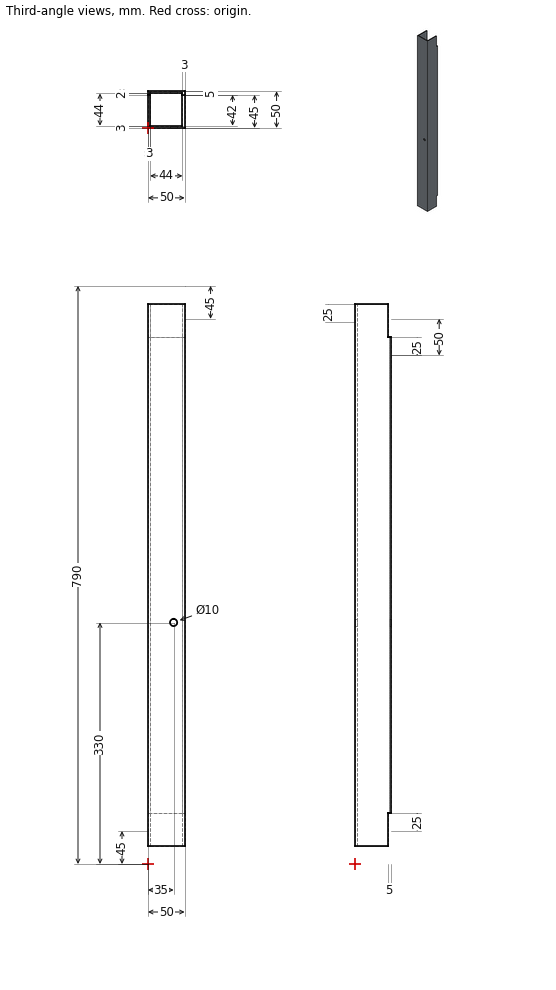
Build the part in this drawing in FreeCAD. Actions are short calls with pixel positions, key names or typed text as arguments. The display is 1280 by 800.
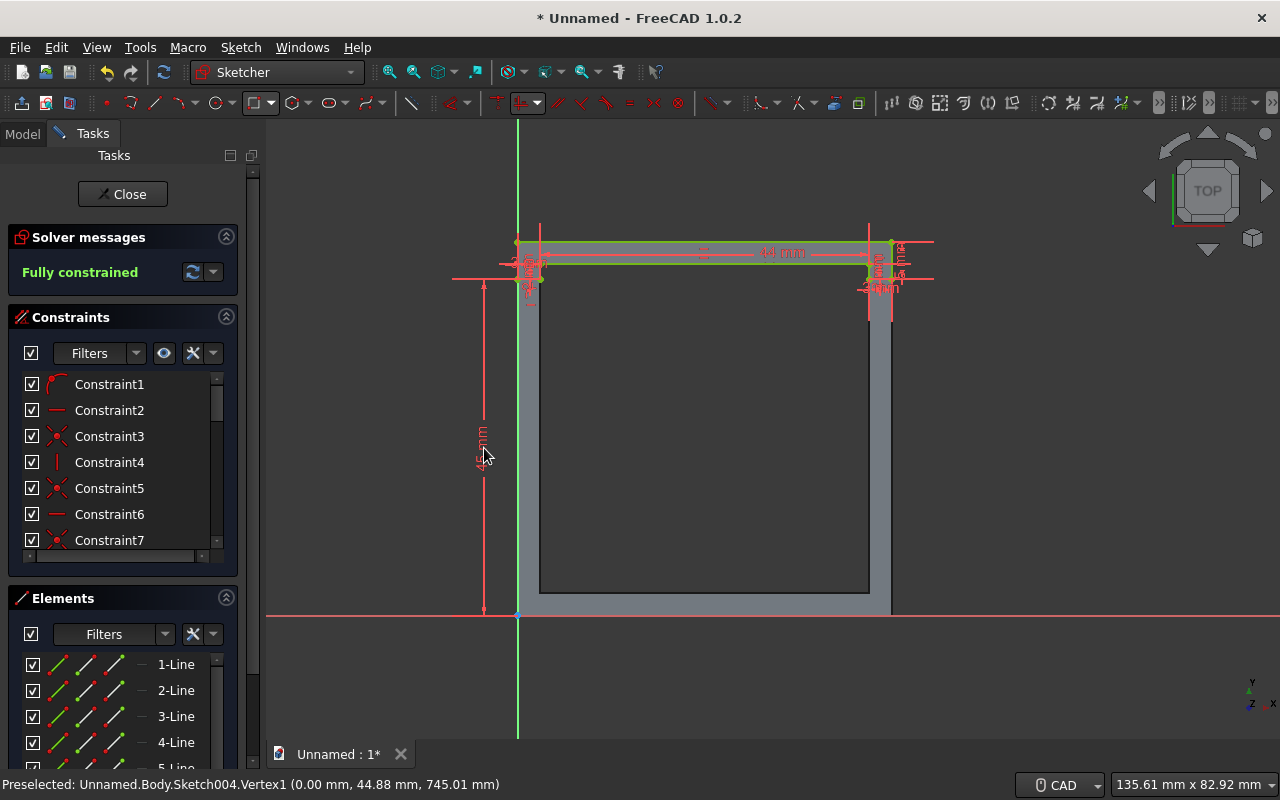
click(123, 194)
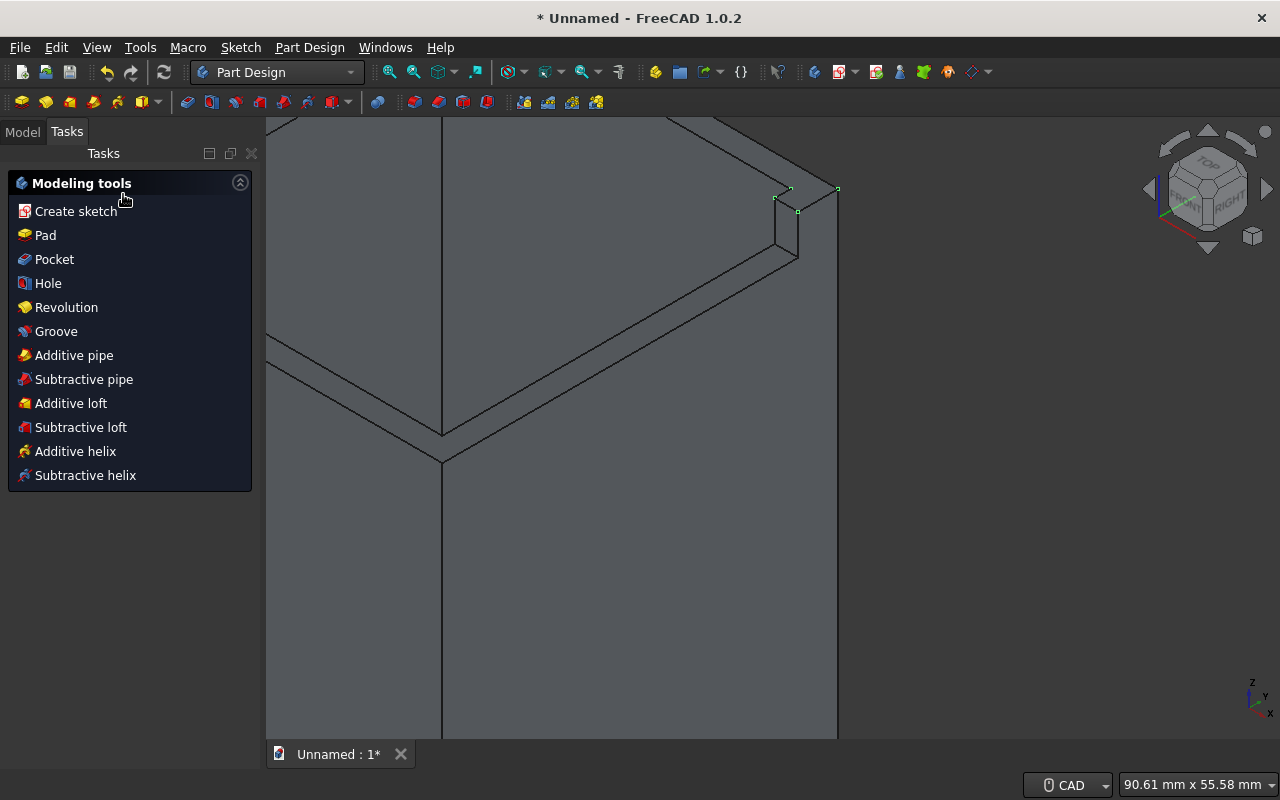
click(188, 102)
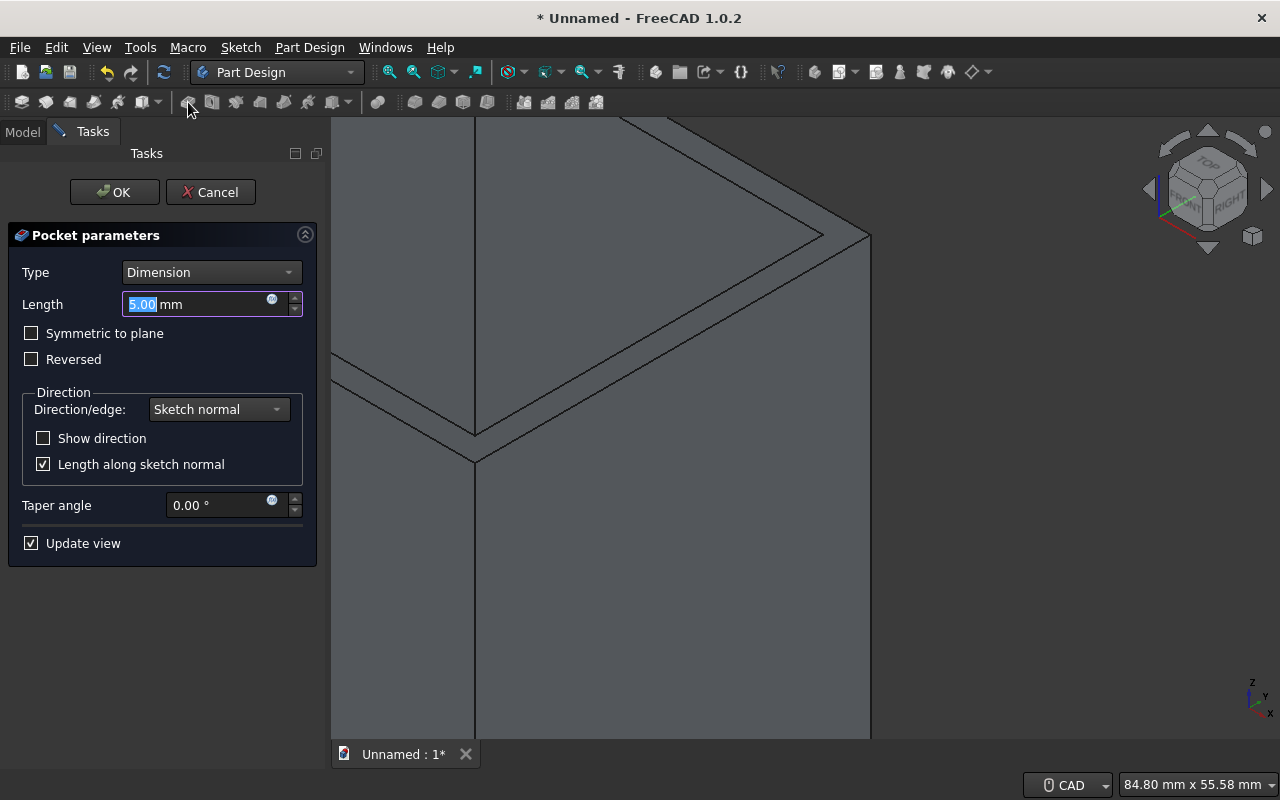
text(50)
key(Tab)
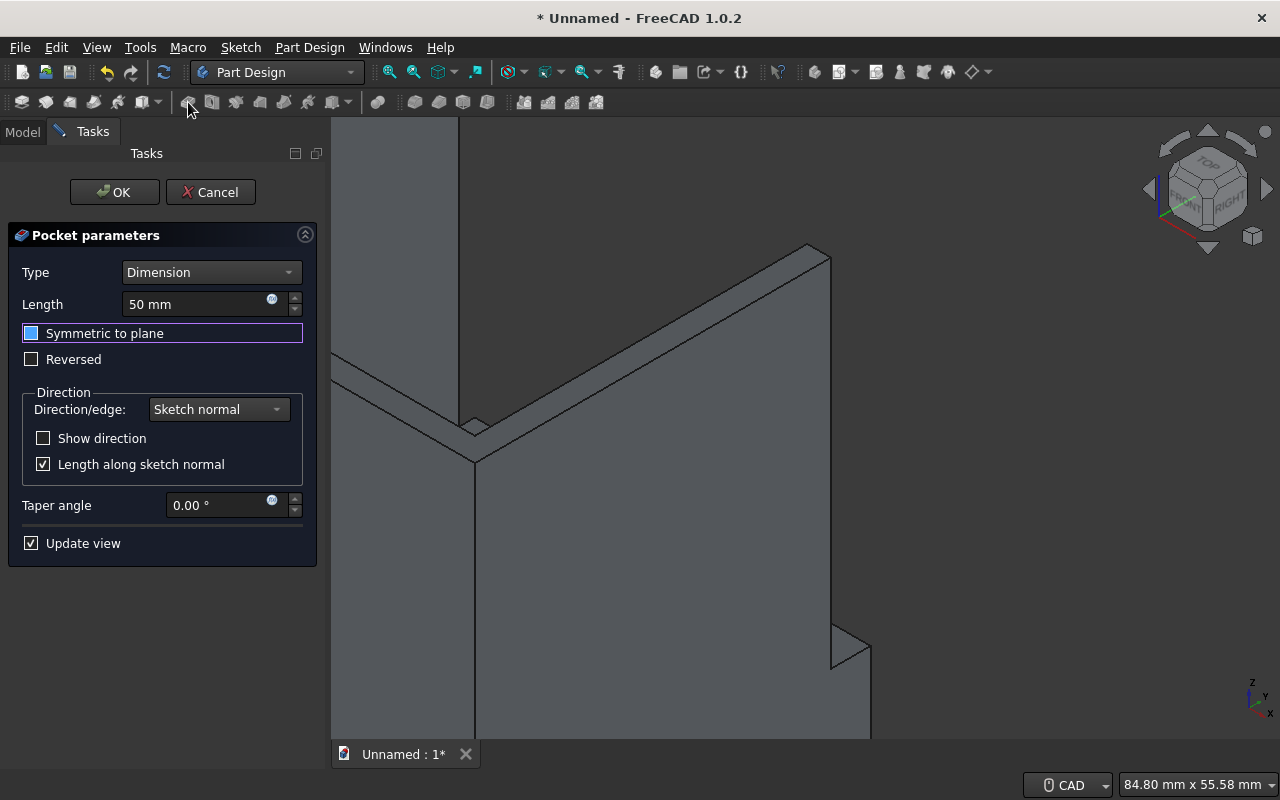
click(115, 192)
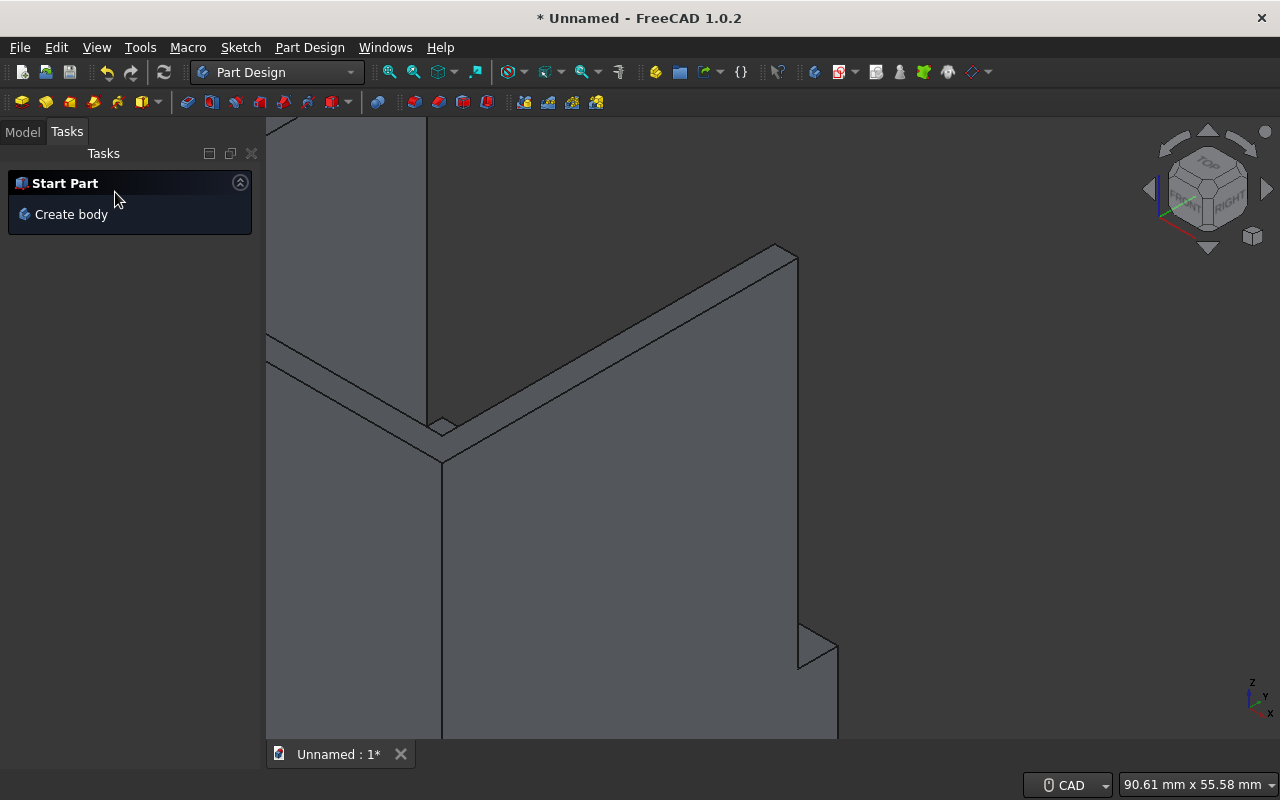
click(390, 72)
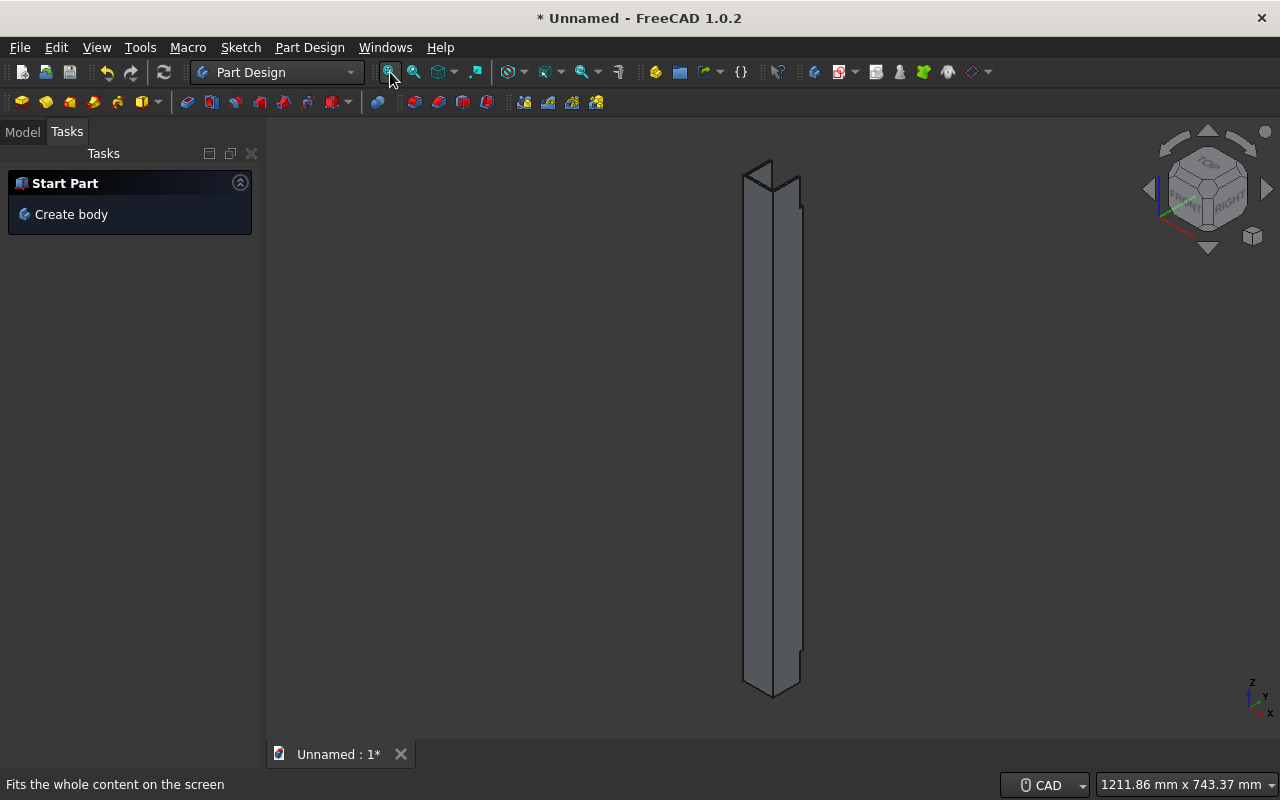
scroll(799, 204, up, 13)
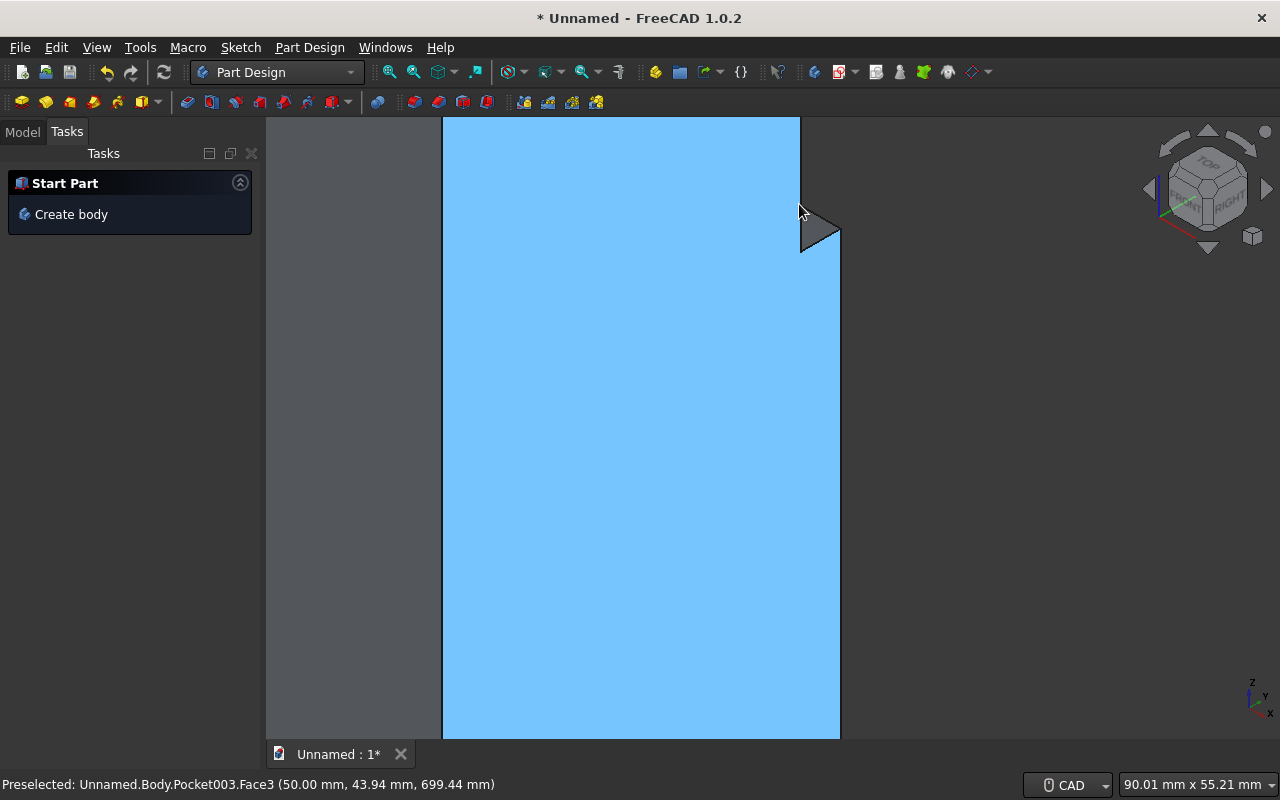
click(390, 72)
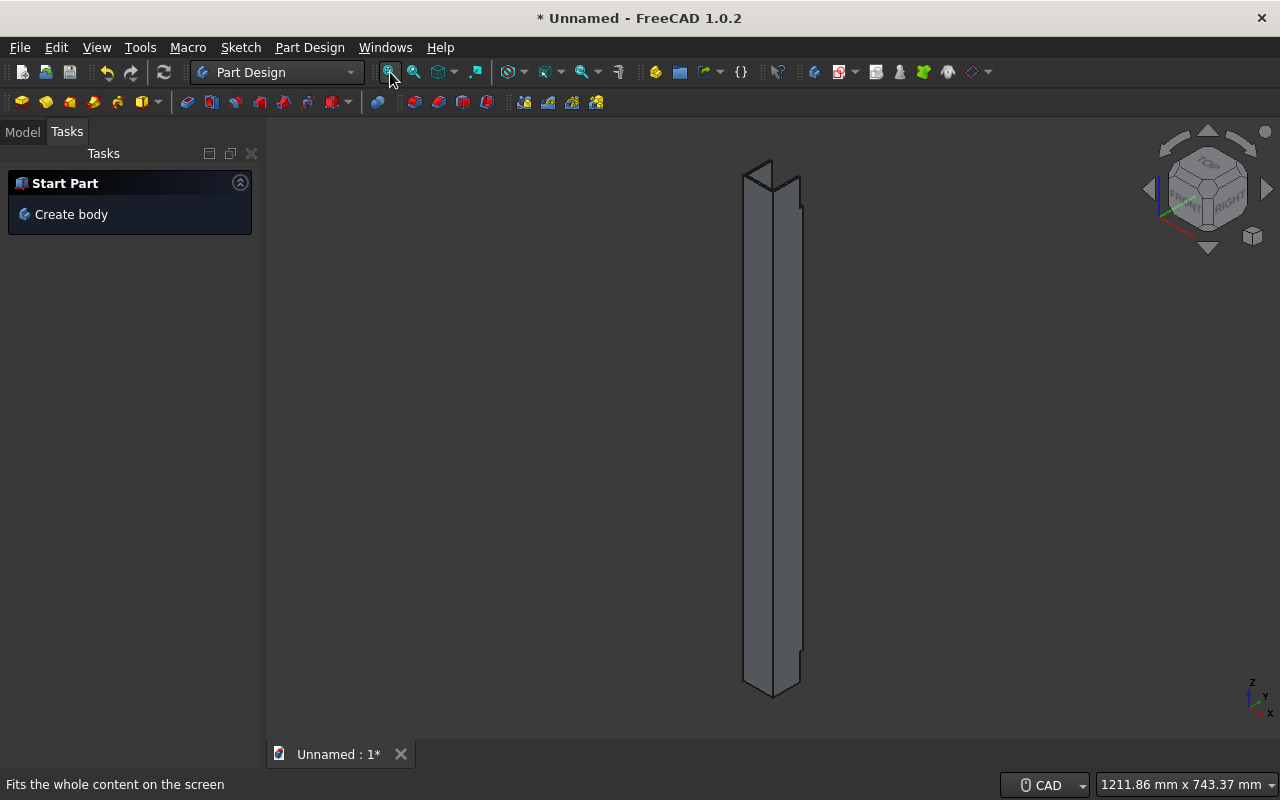
key(2)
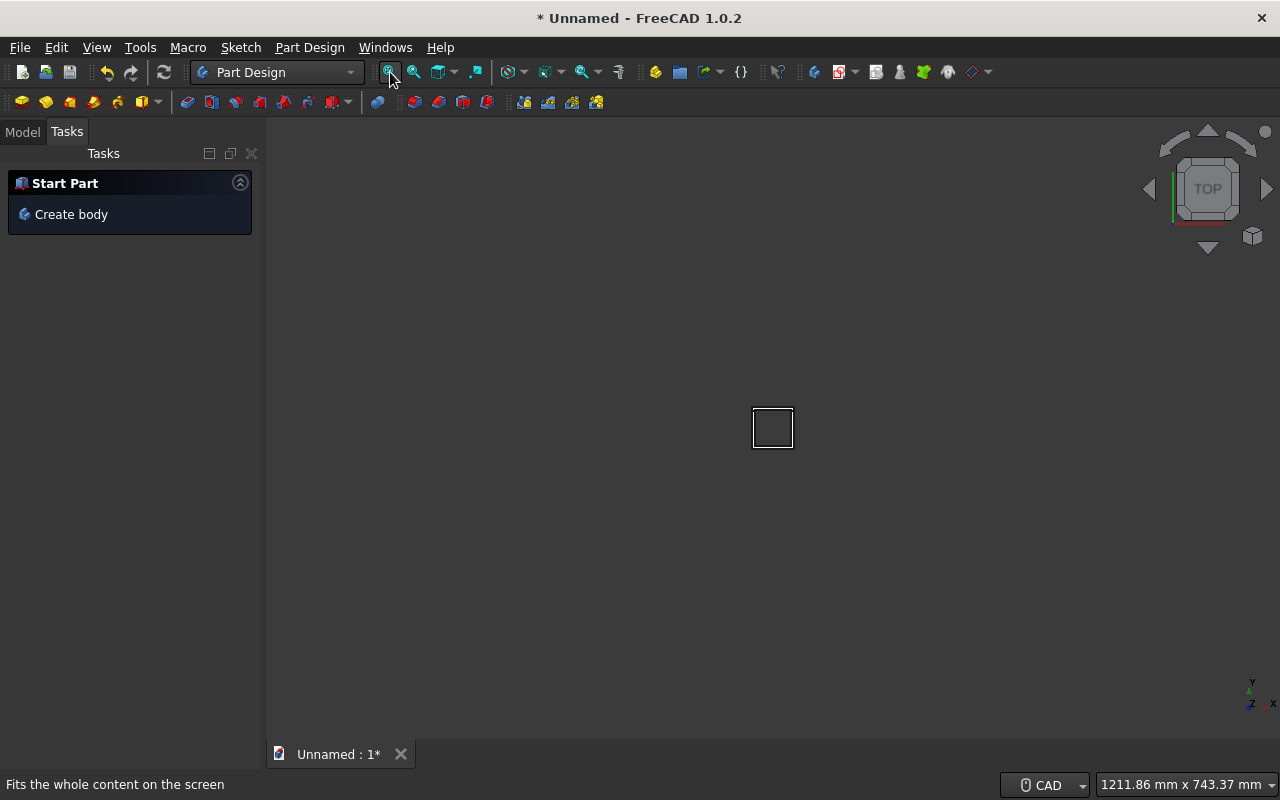
click(390, 72)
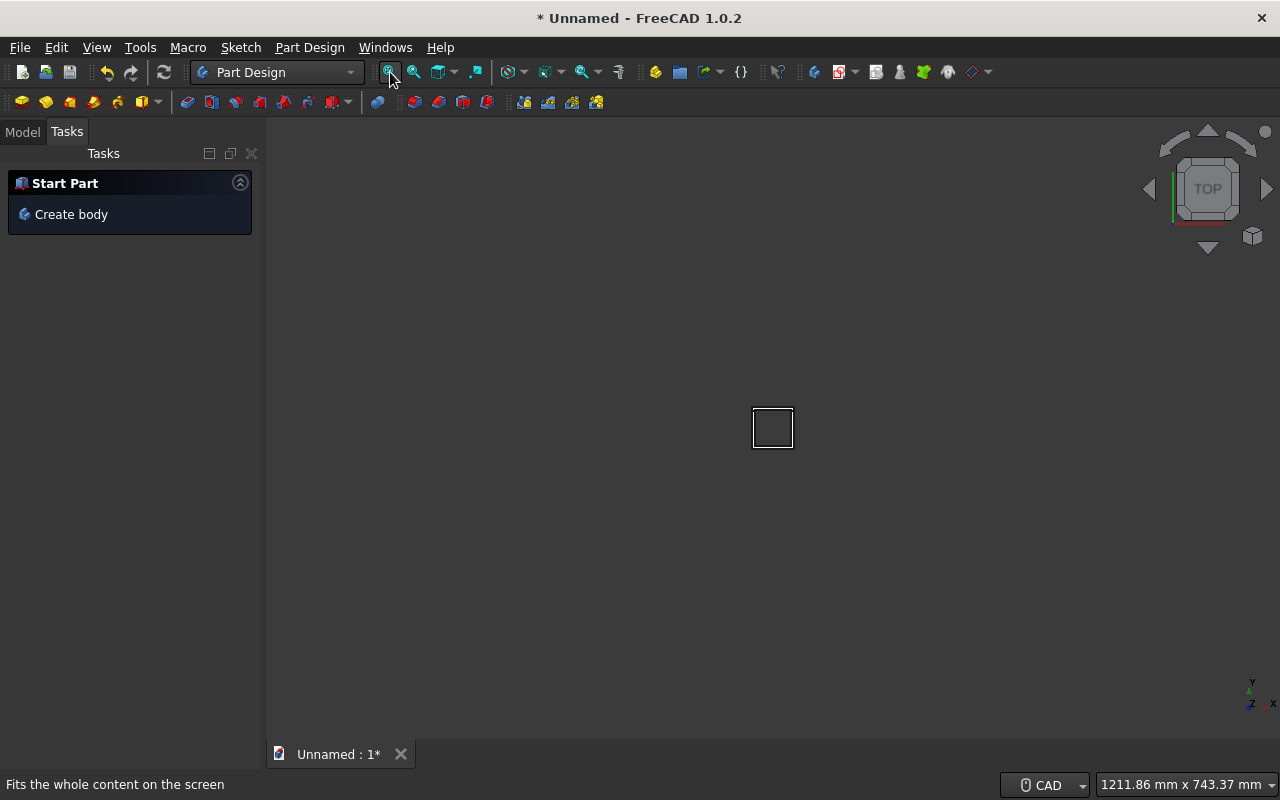
scroll(791, 408, up, 13)